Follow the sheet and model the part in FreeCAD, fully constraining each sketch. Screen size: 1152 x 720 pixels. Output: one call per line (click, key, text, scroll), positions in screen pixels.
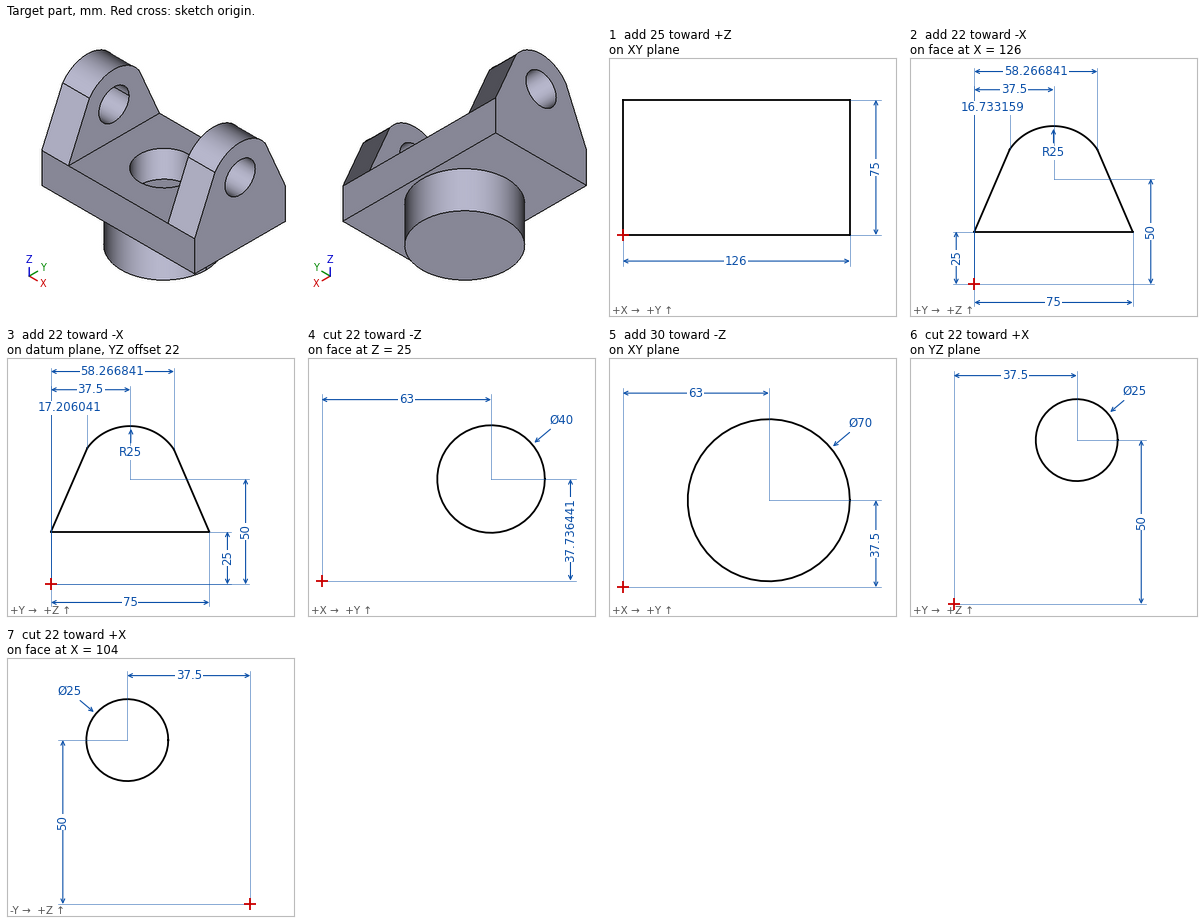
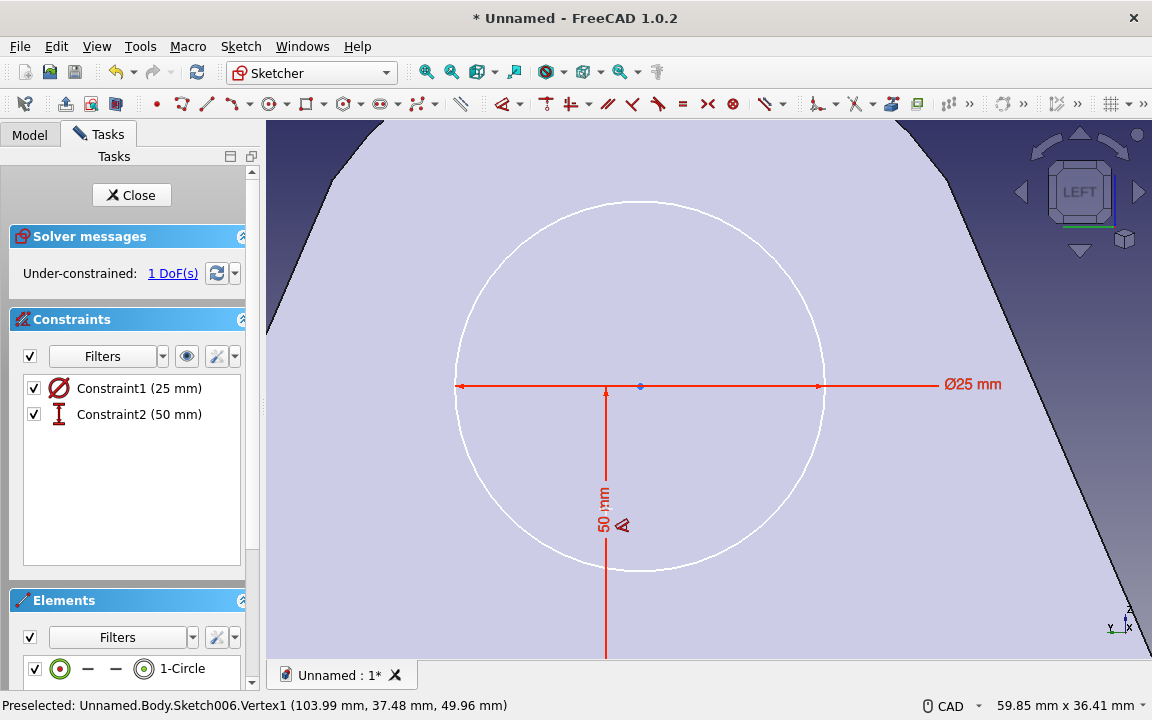
click(640, 386)
click(734, 352)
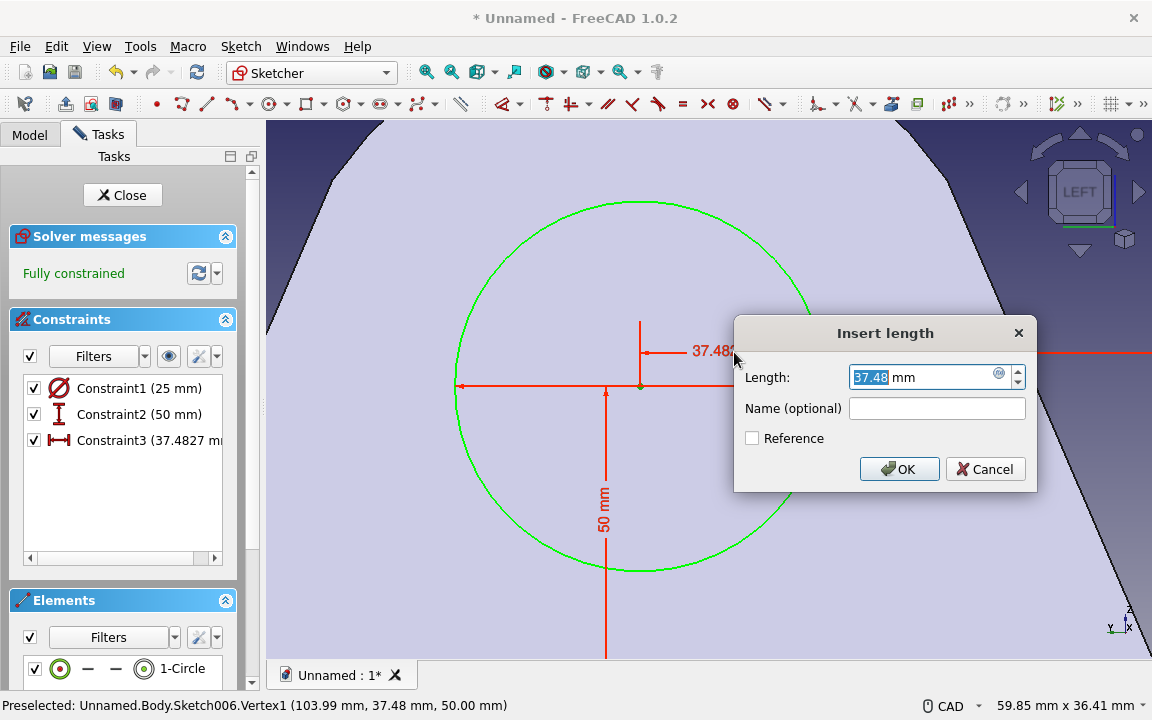
text(37.5)
key(Return)
key(Escape)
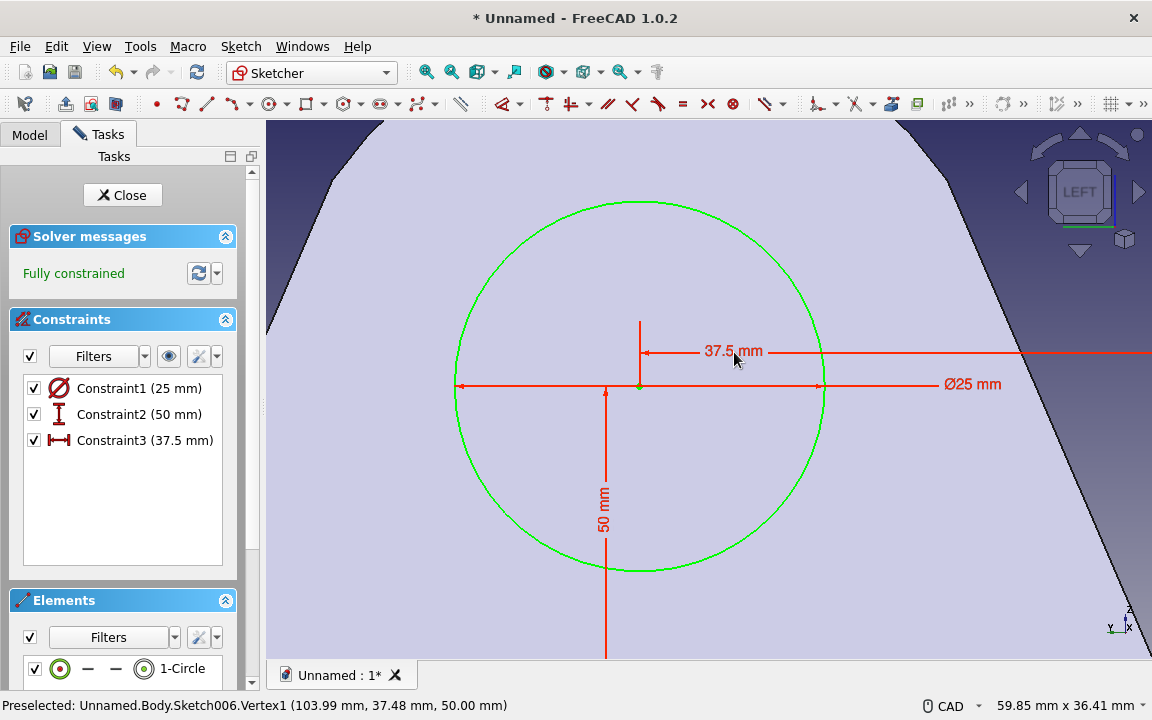
click(123, 195)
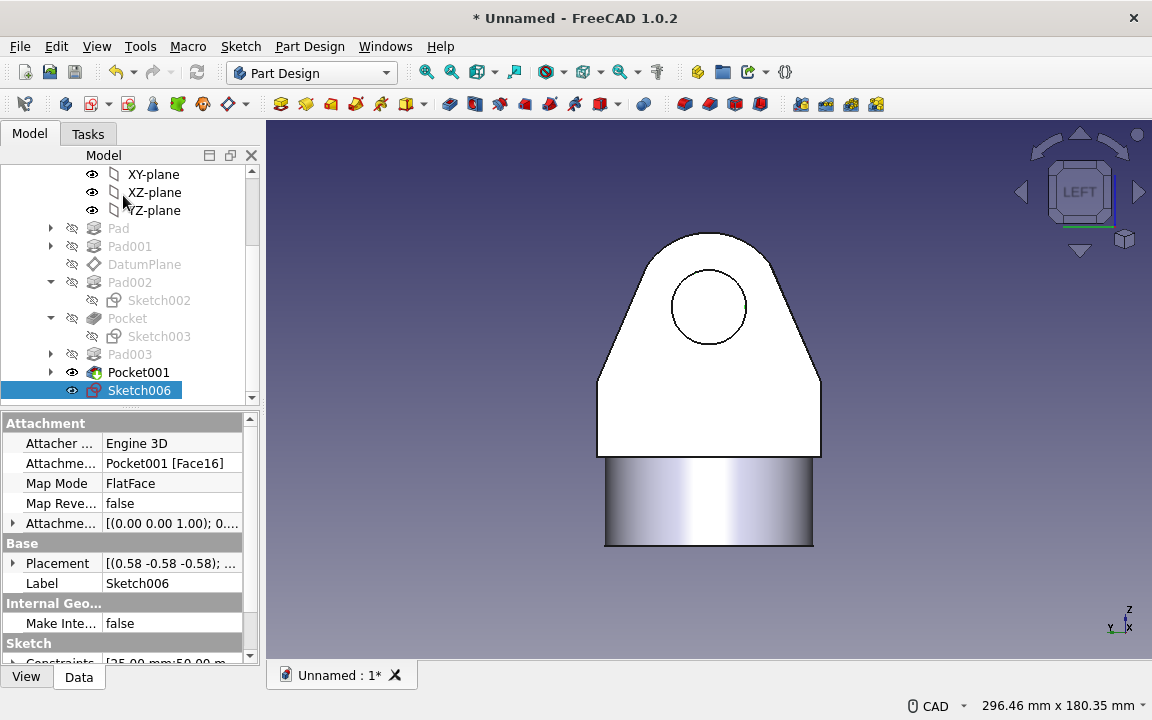
click(450, 104)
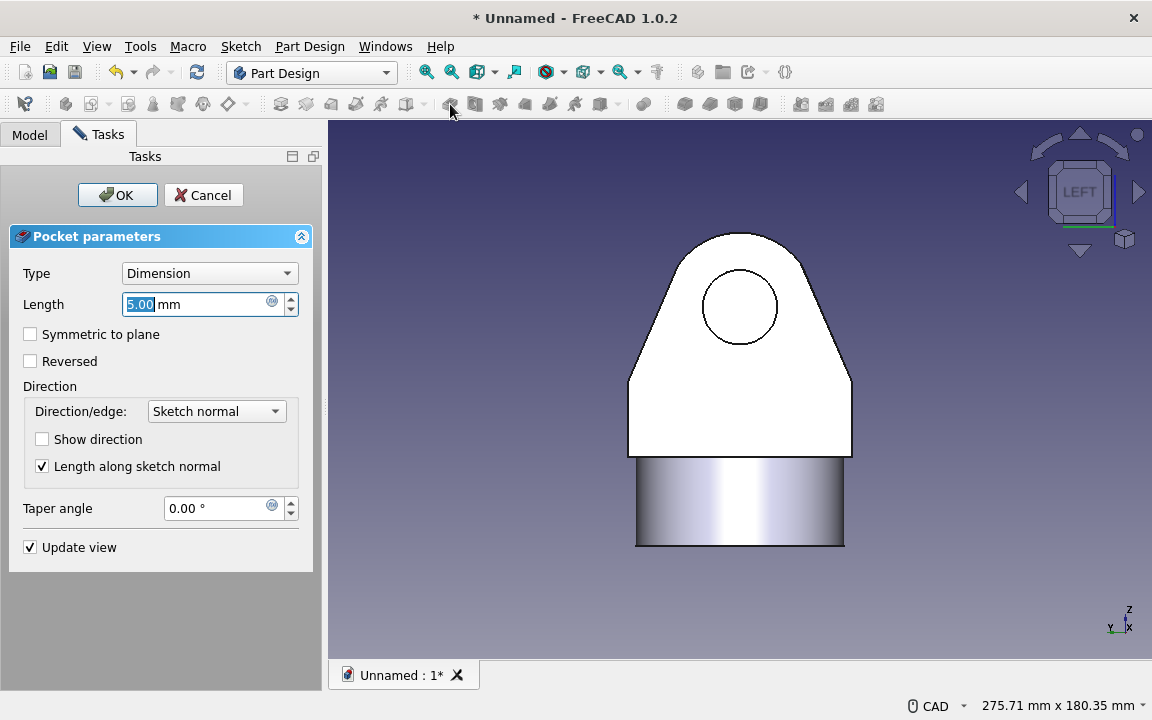
text(22)
key(Tab)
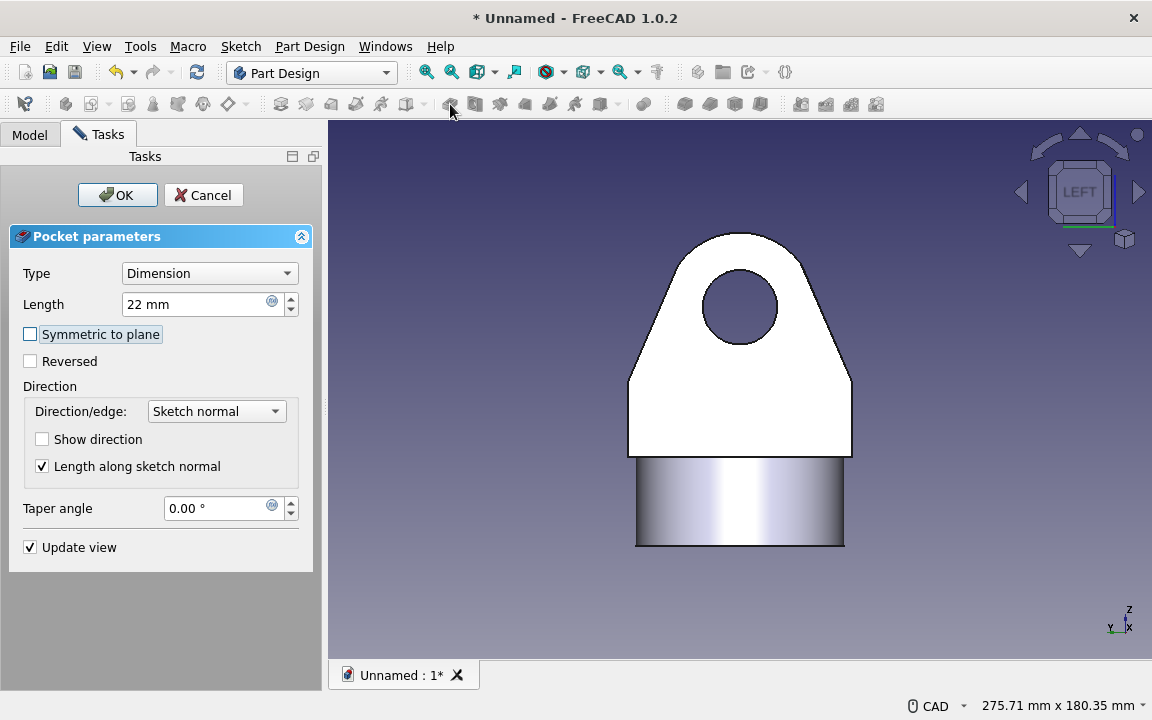
click(118, 195)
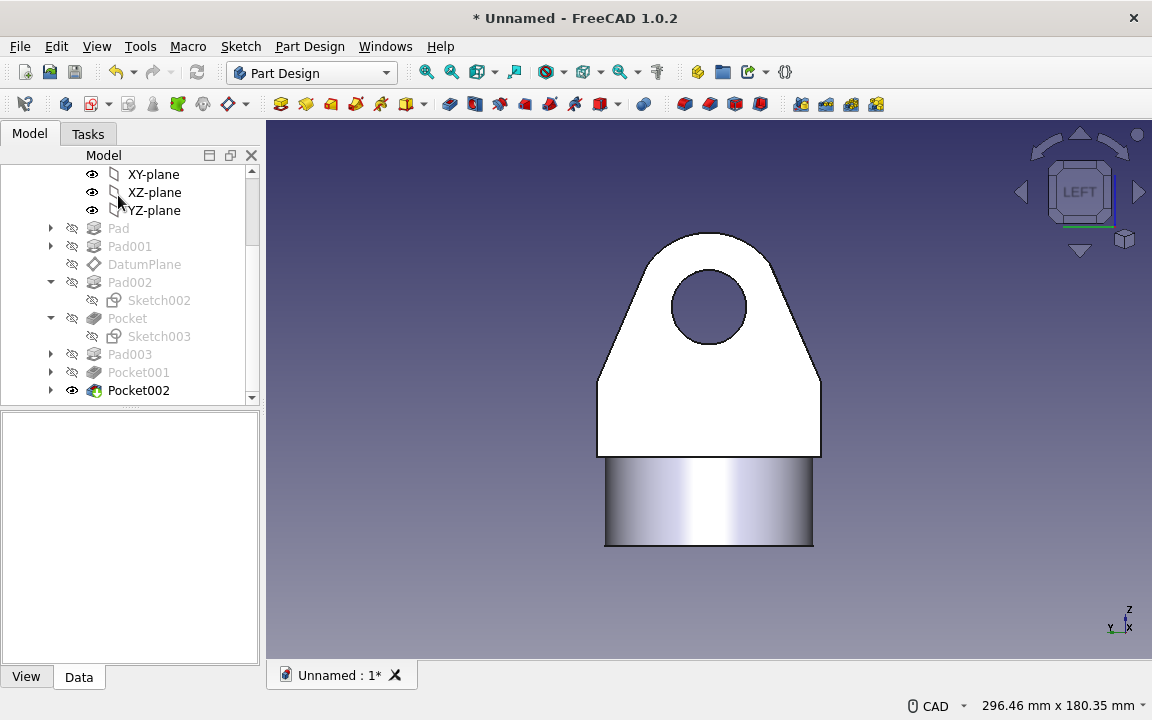
key(0)